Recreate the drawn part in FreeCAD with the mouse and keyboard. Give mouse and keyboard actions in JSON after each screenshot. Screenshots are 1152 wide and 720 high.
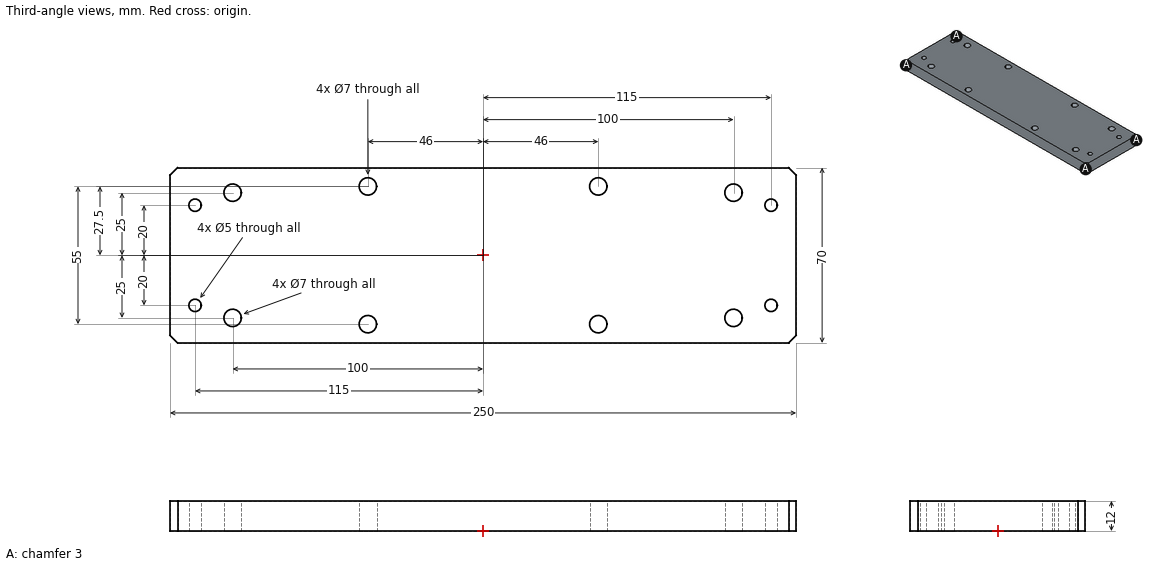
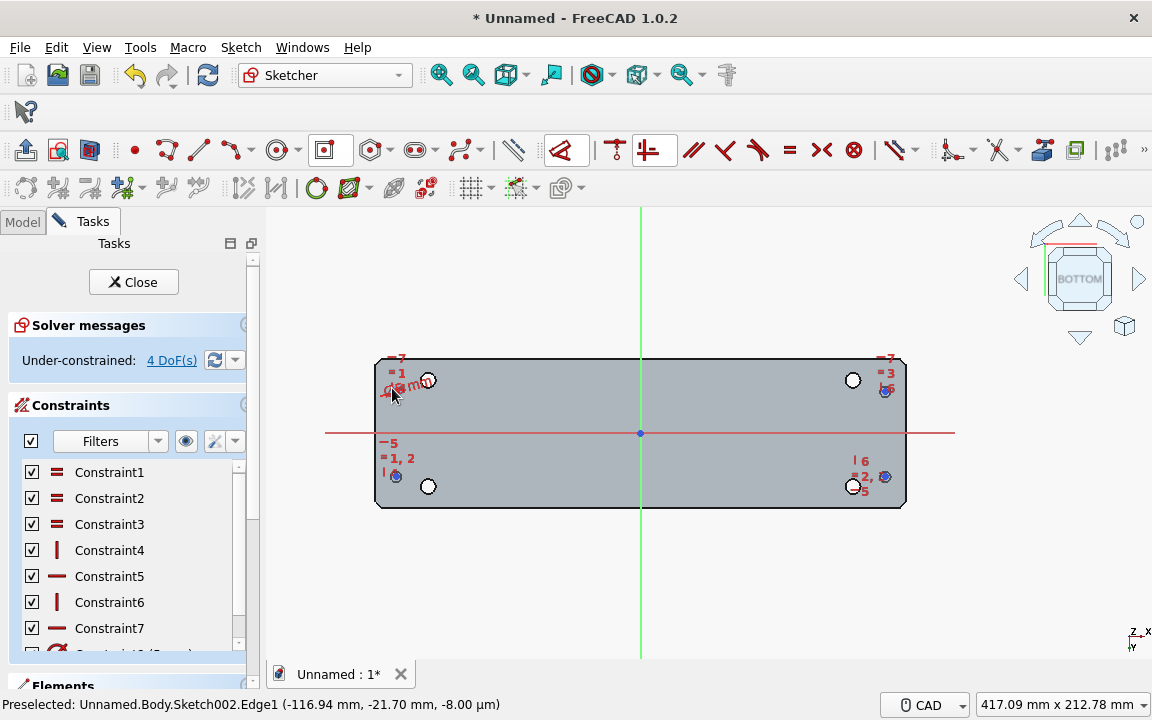
{"action": "left_click", "coordinate": [396, 392]}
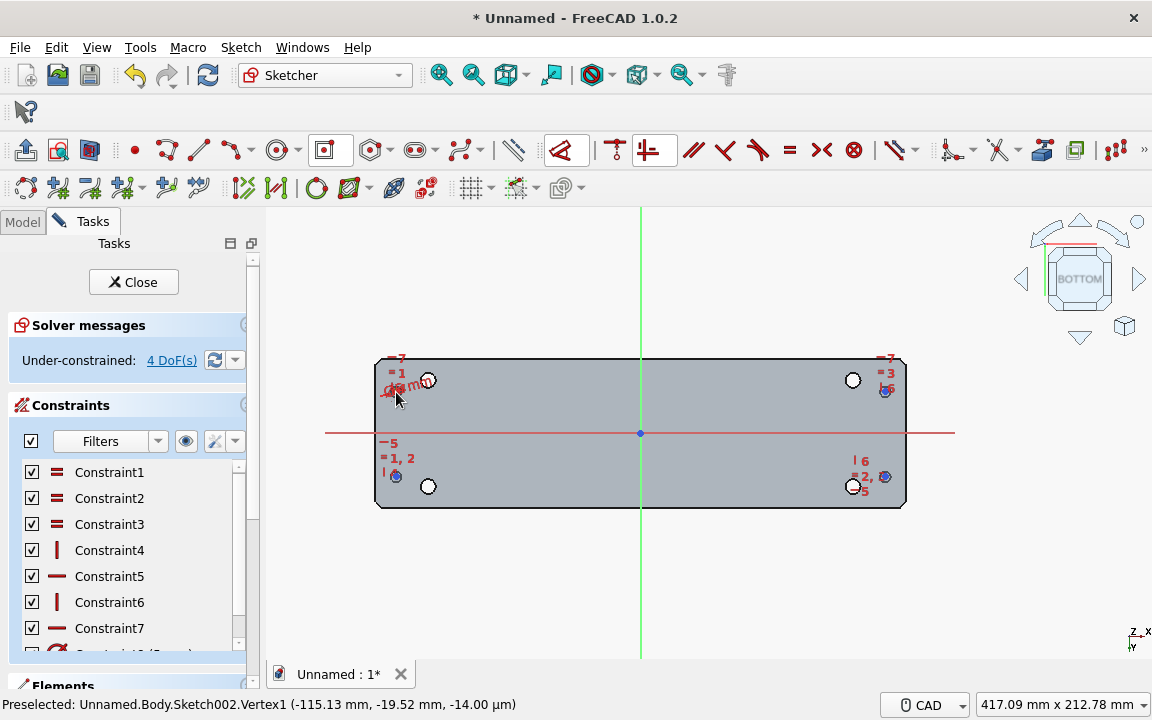
{"action": "left_click", "coordinate": [584, 150]}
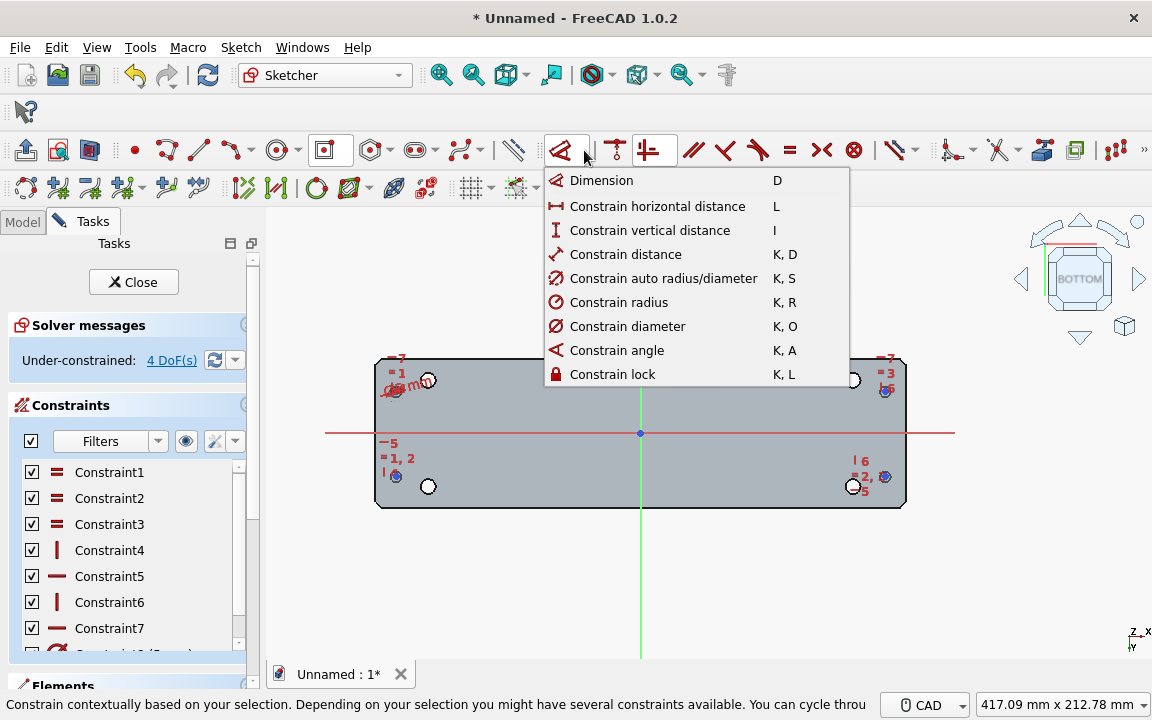
{"action": "left_click", "coordinate": [697, 230]}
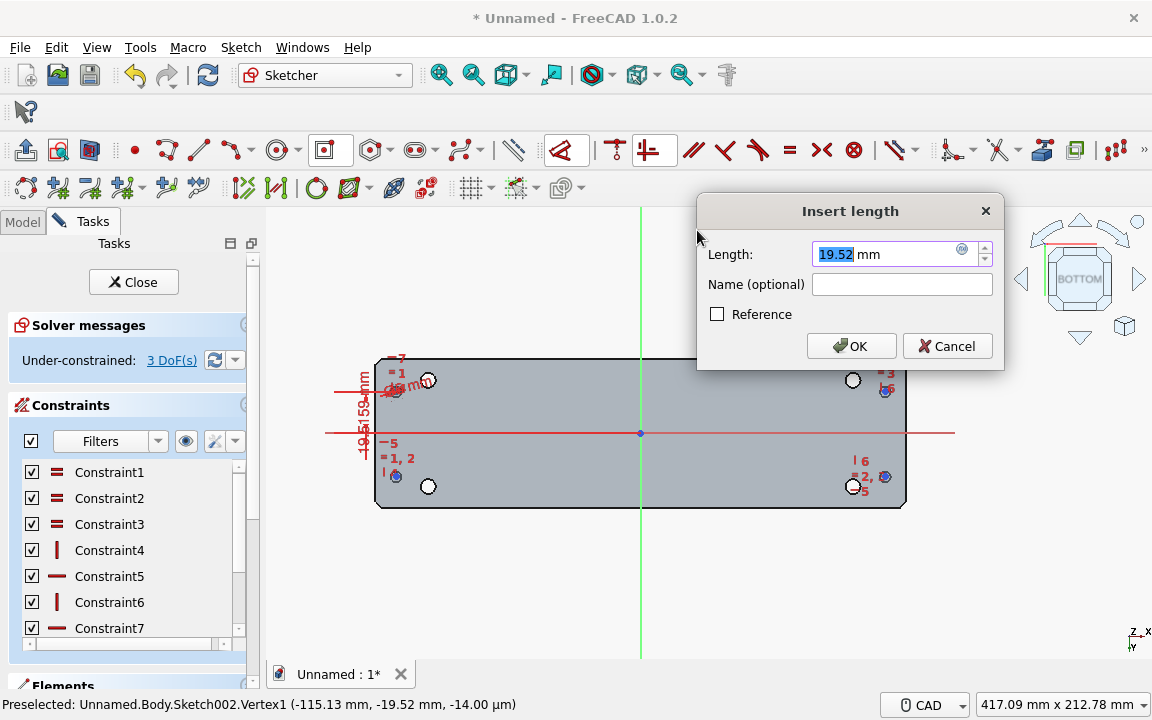
{"action": "type", "text": "20"}
{"action": "key", "text": "Return"}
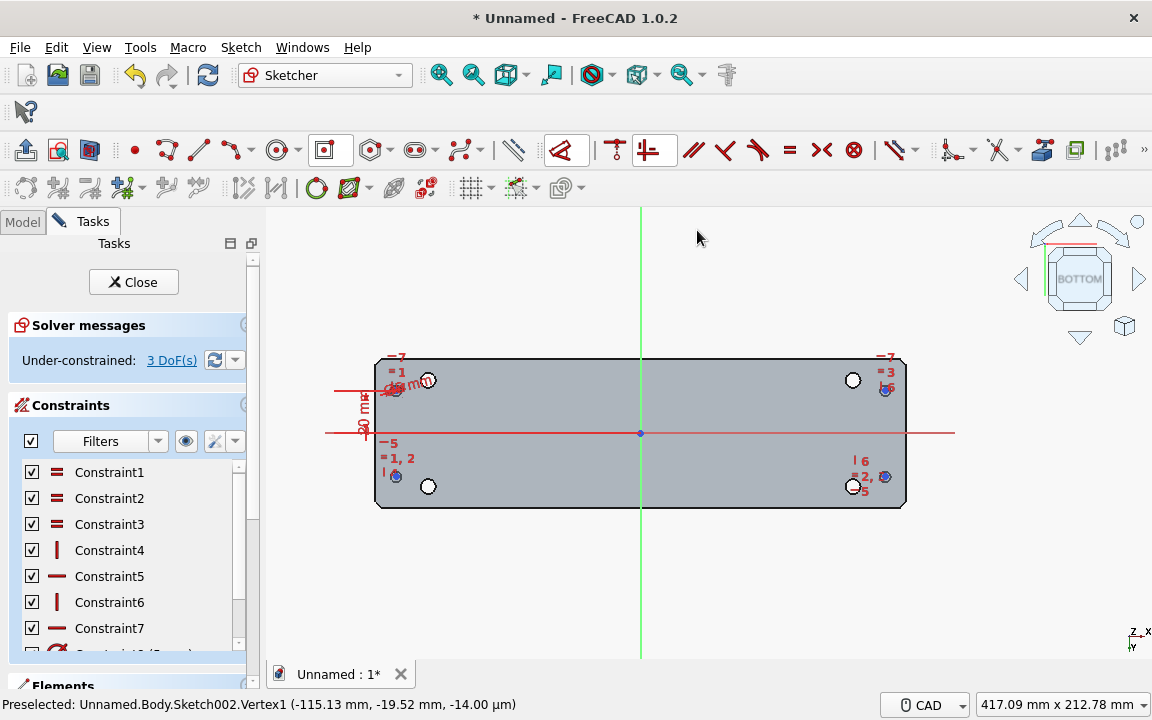
{"action": "left_click", "coordinate": [396, 477]}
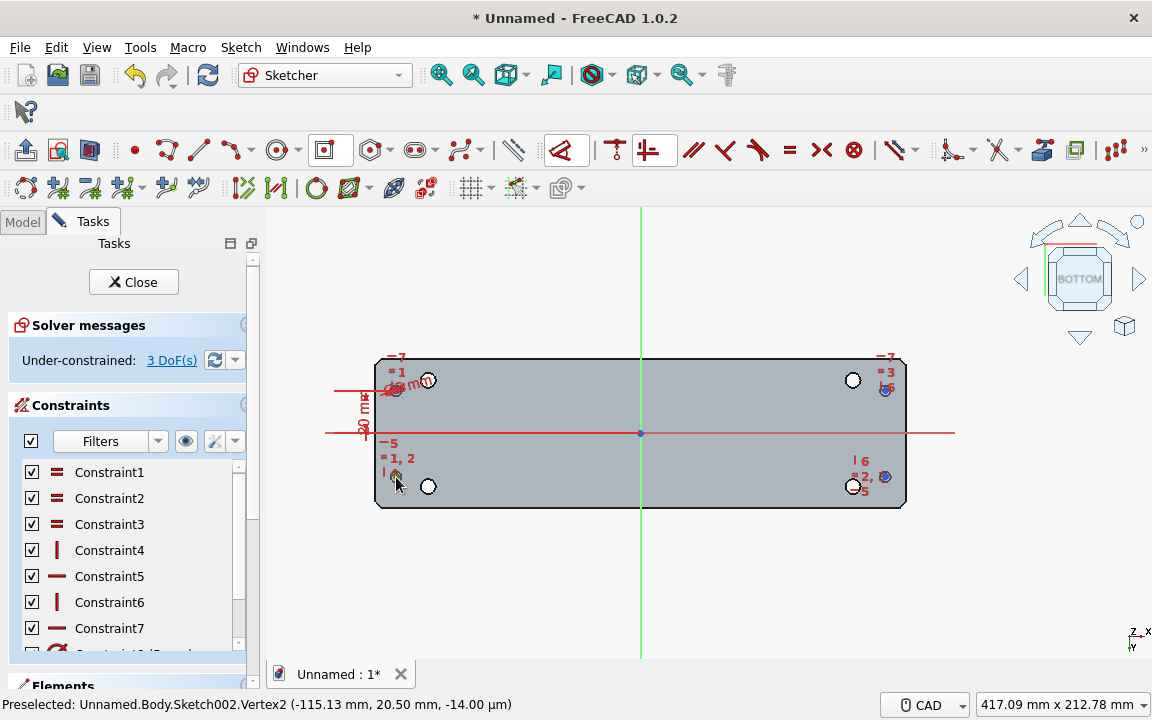
{"action": "key", "text": "i"}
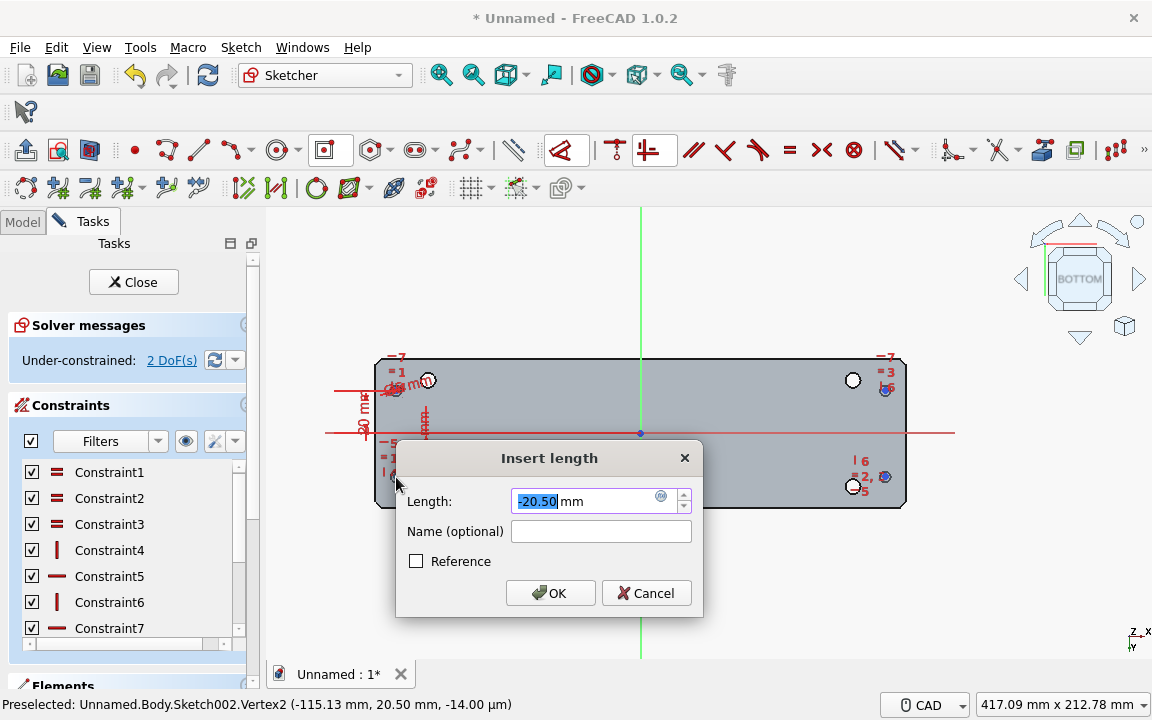
{"action": "type", "text": "-20"}
{"action": "key", "text": "Return"}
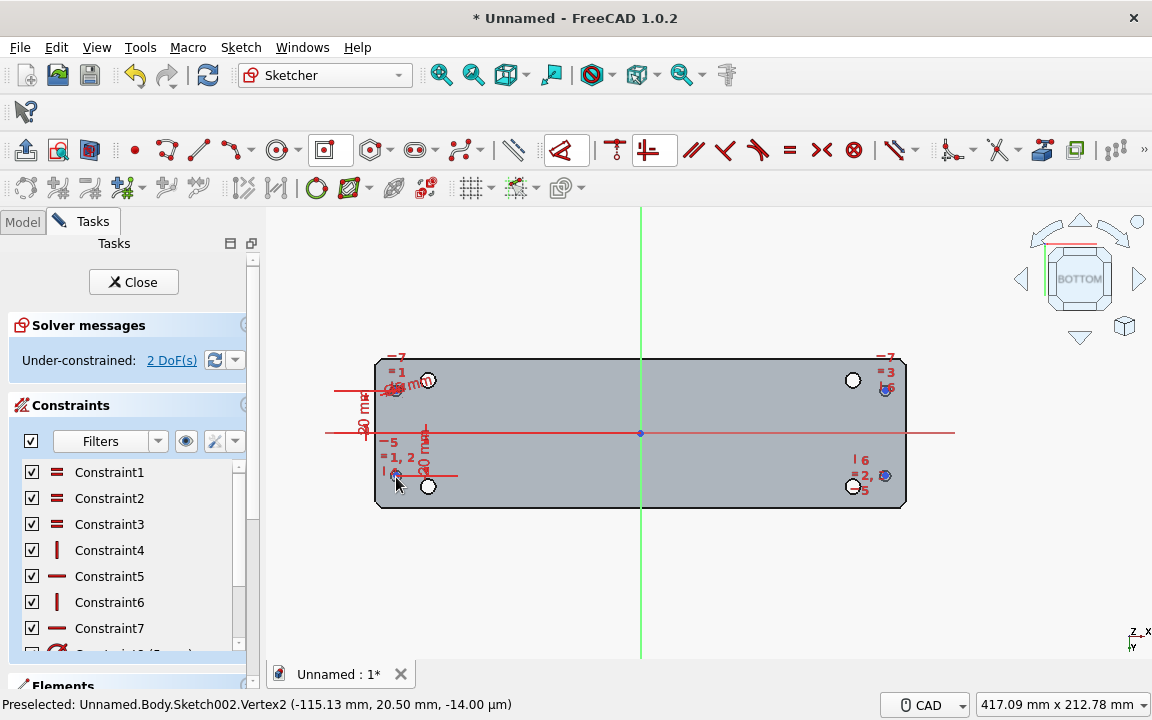
{"action": "left_click", "coordinate": [396, 391]}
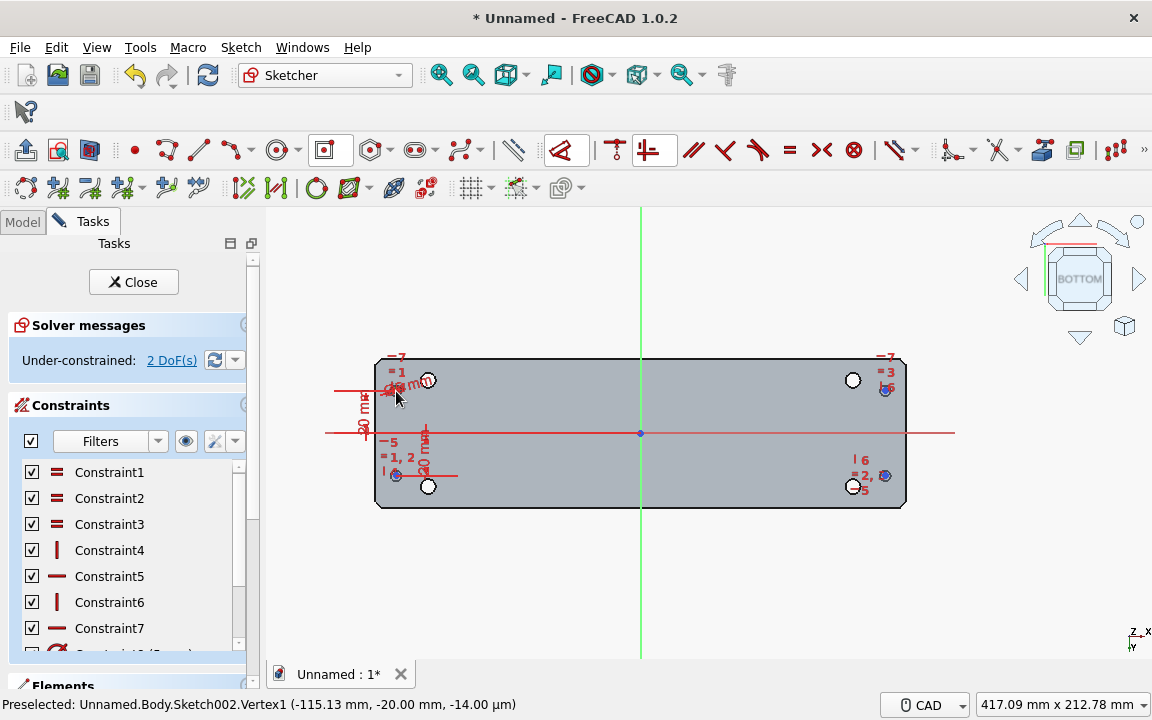
{"action": "left_click", "coordinate": [584, 150]}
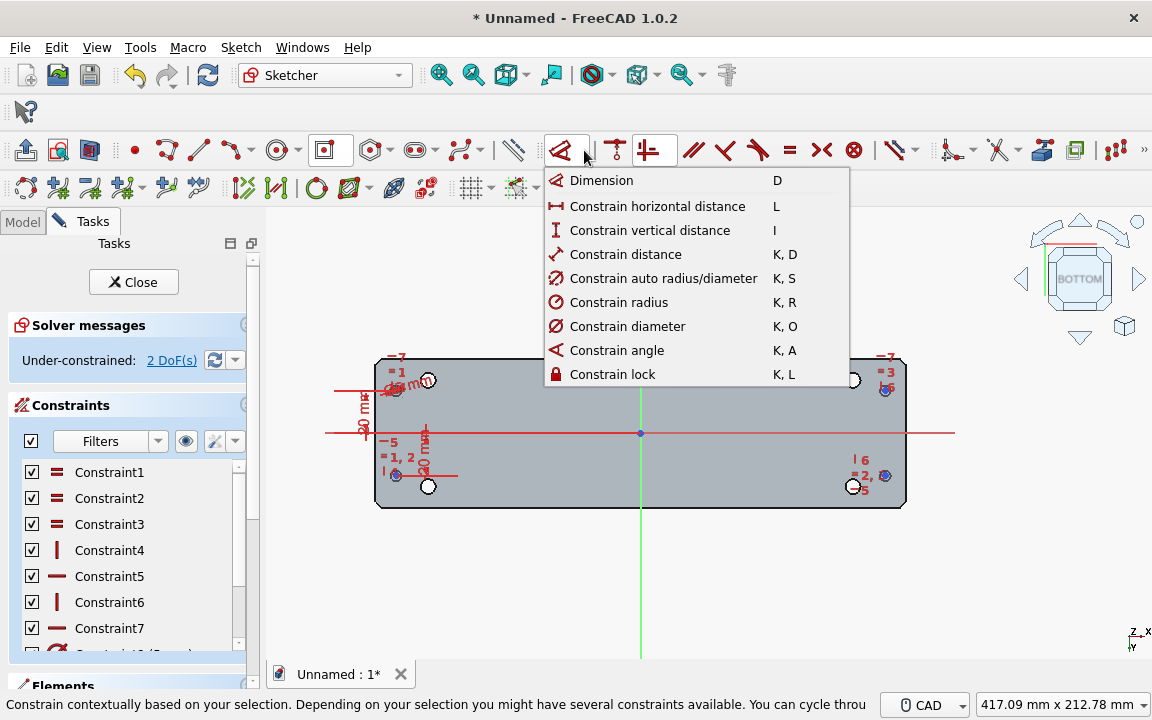
{"action": "left_click", "coordinate": [697, 206]}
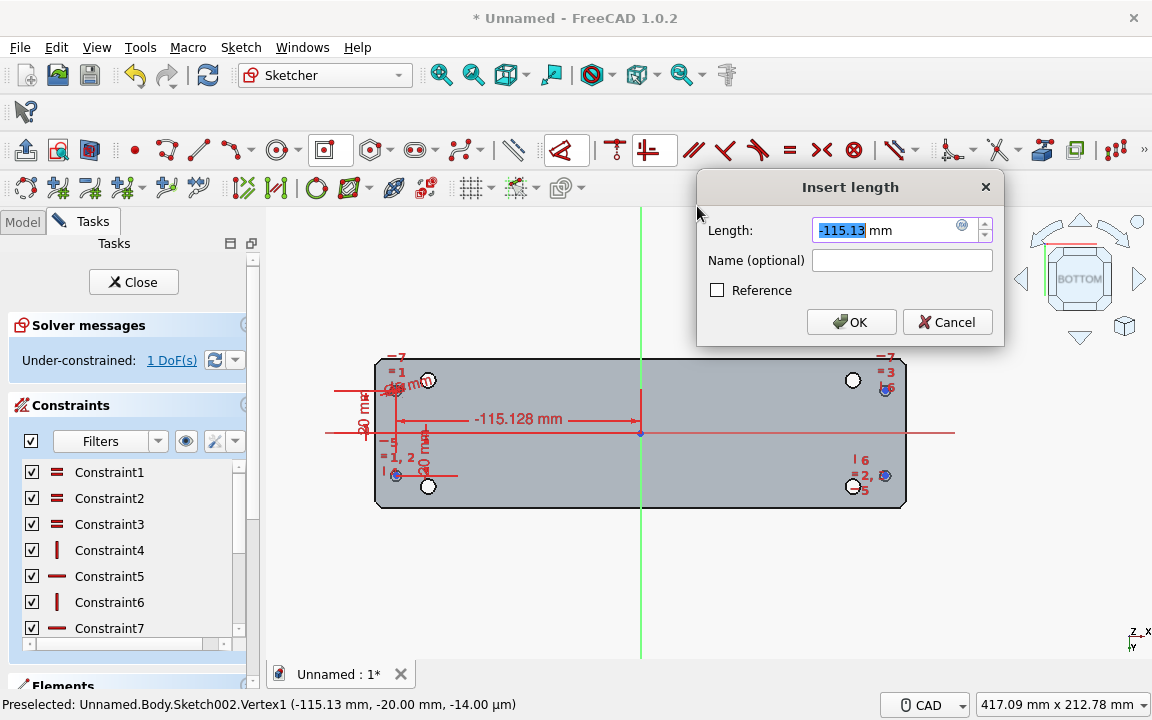
{"action": "type", "text": "-115"}
{"action": "key", "text": "Return"}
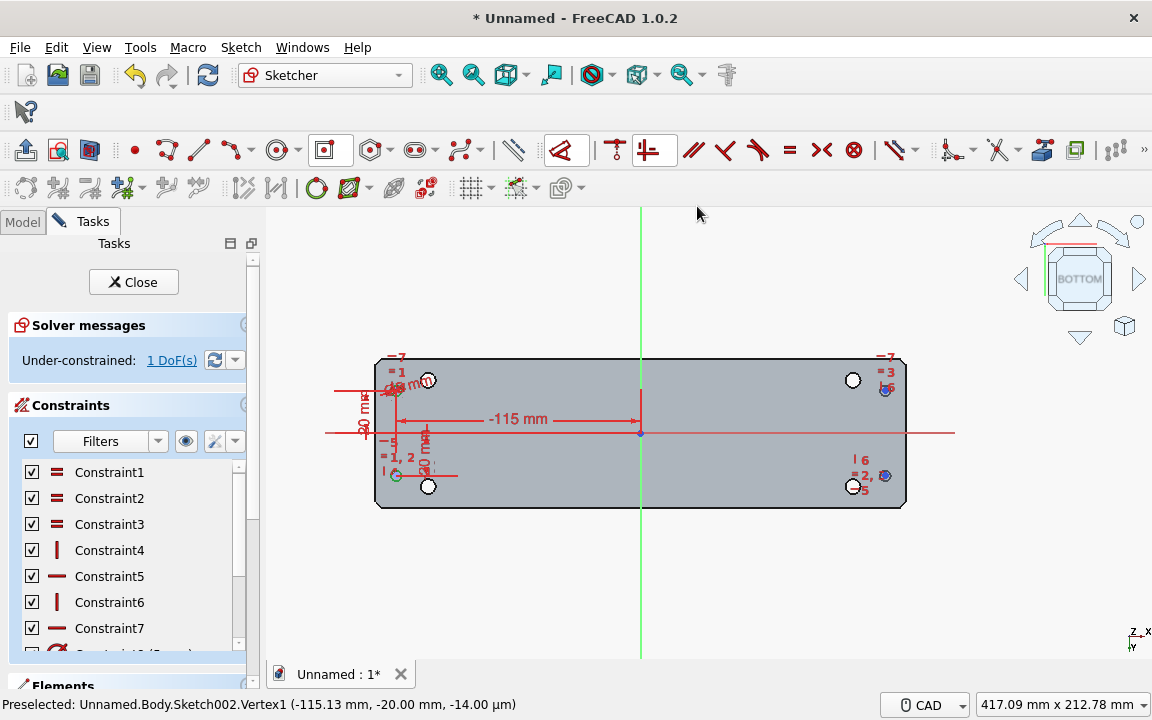
{"action": "left_click", "coordinate": [885, 476]}